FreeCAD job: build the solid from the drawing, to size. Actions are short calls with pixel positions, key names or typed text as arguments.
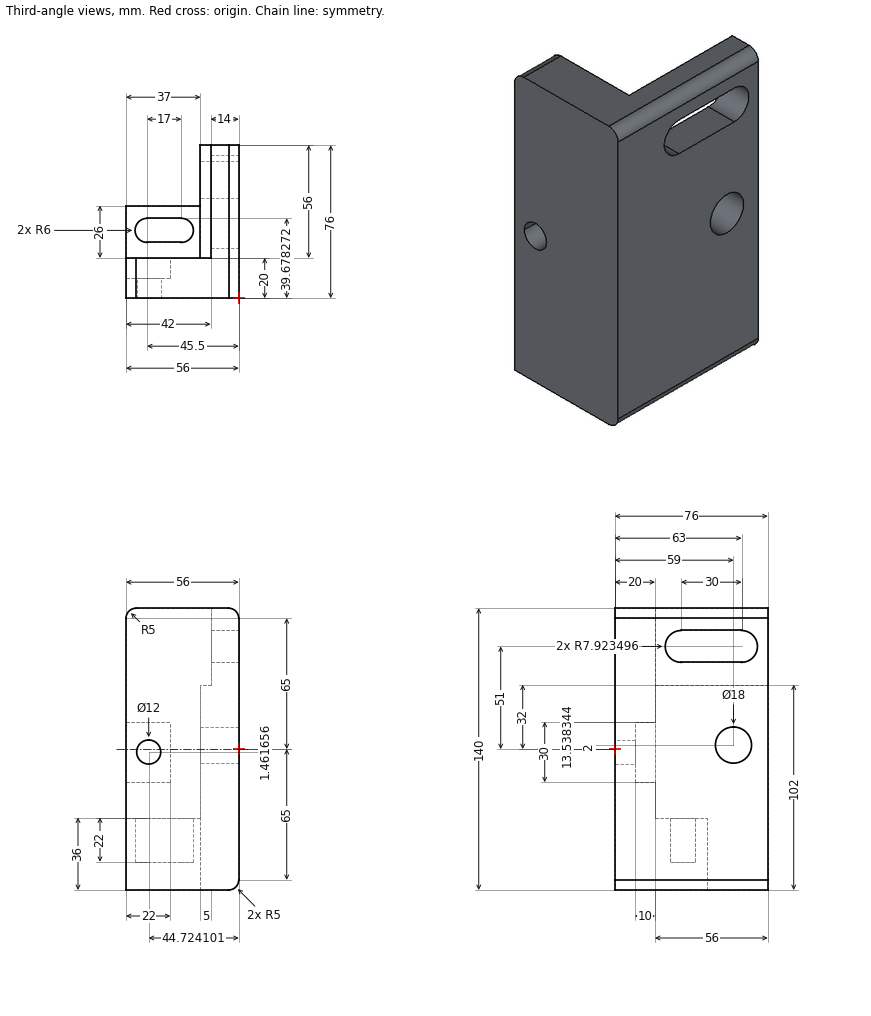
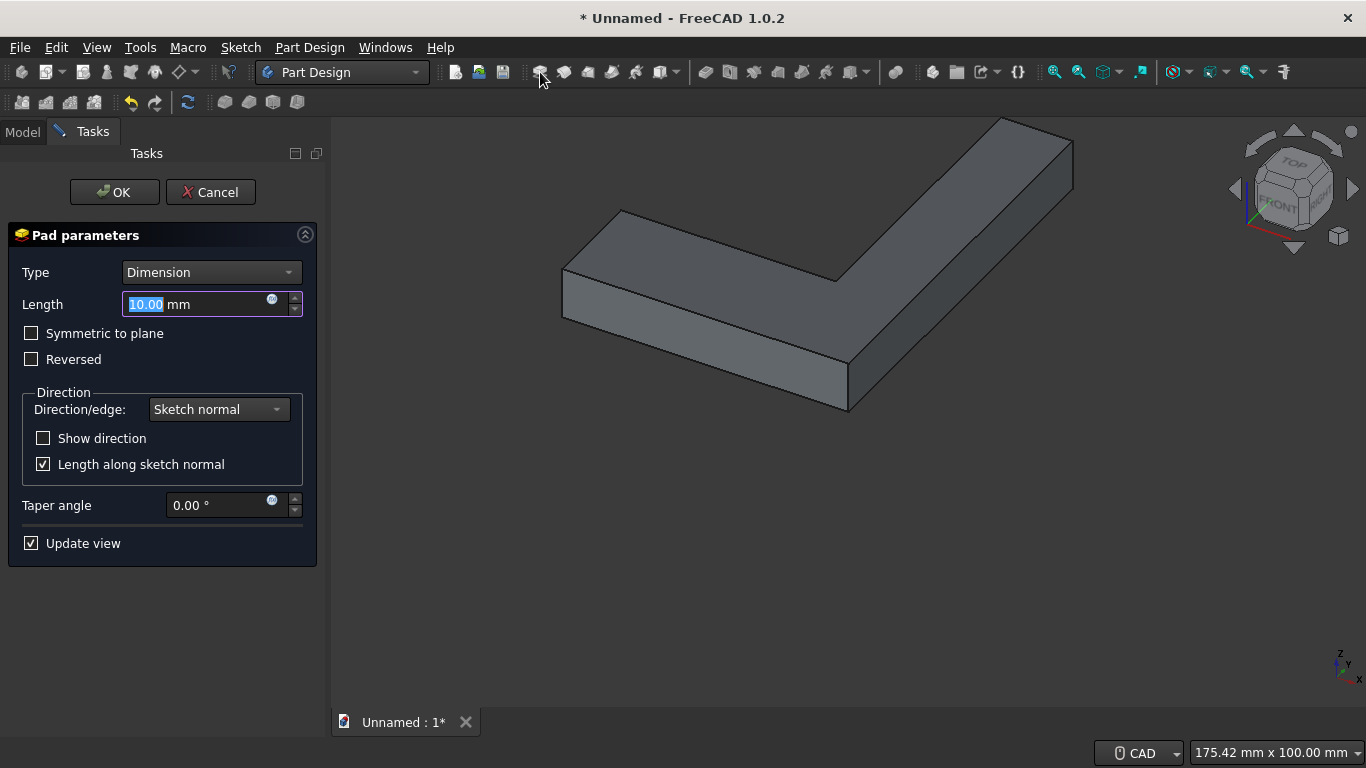
text(140)
key(Tab)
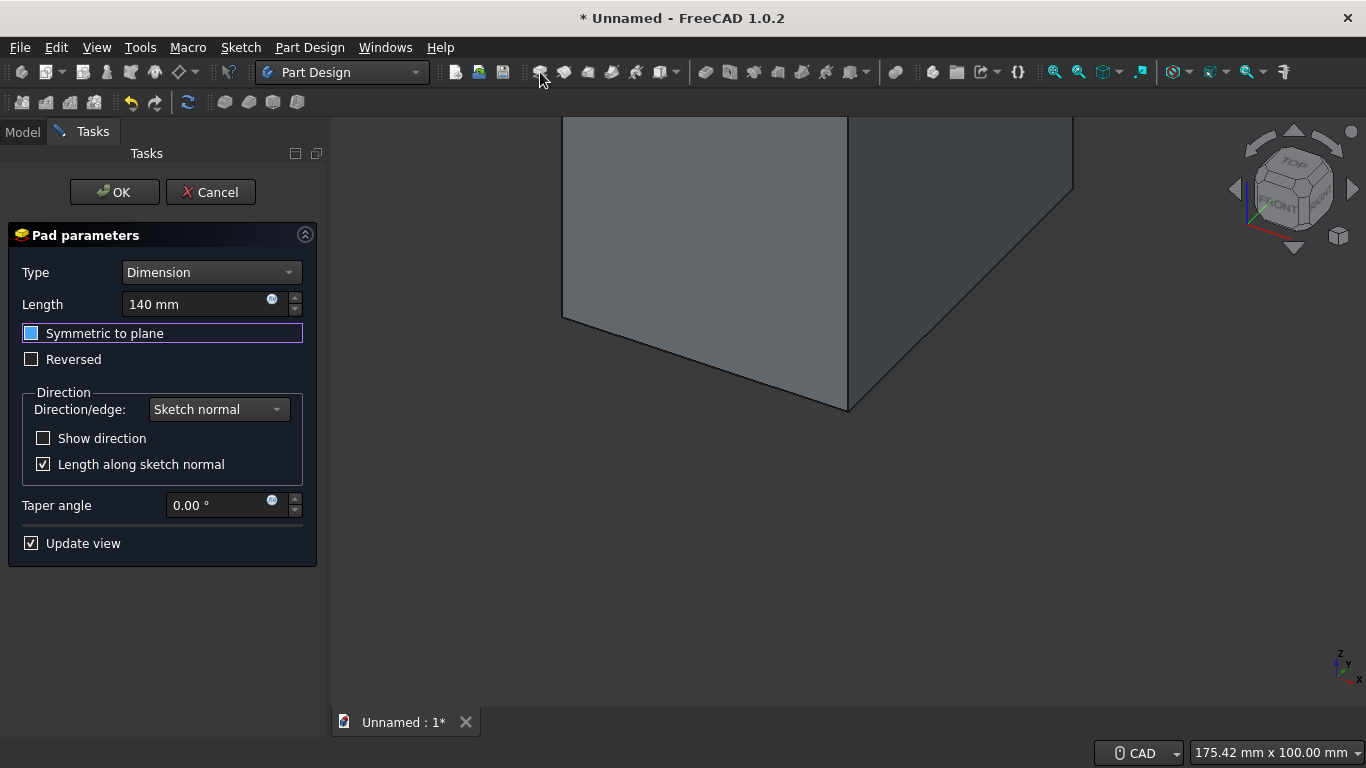
click(30, 333)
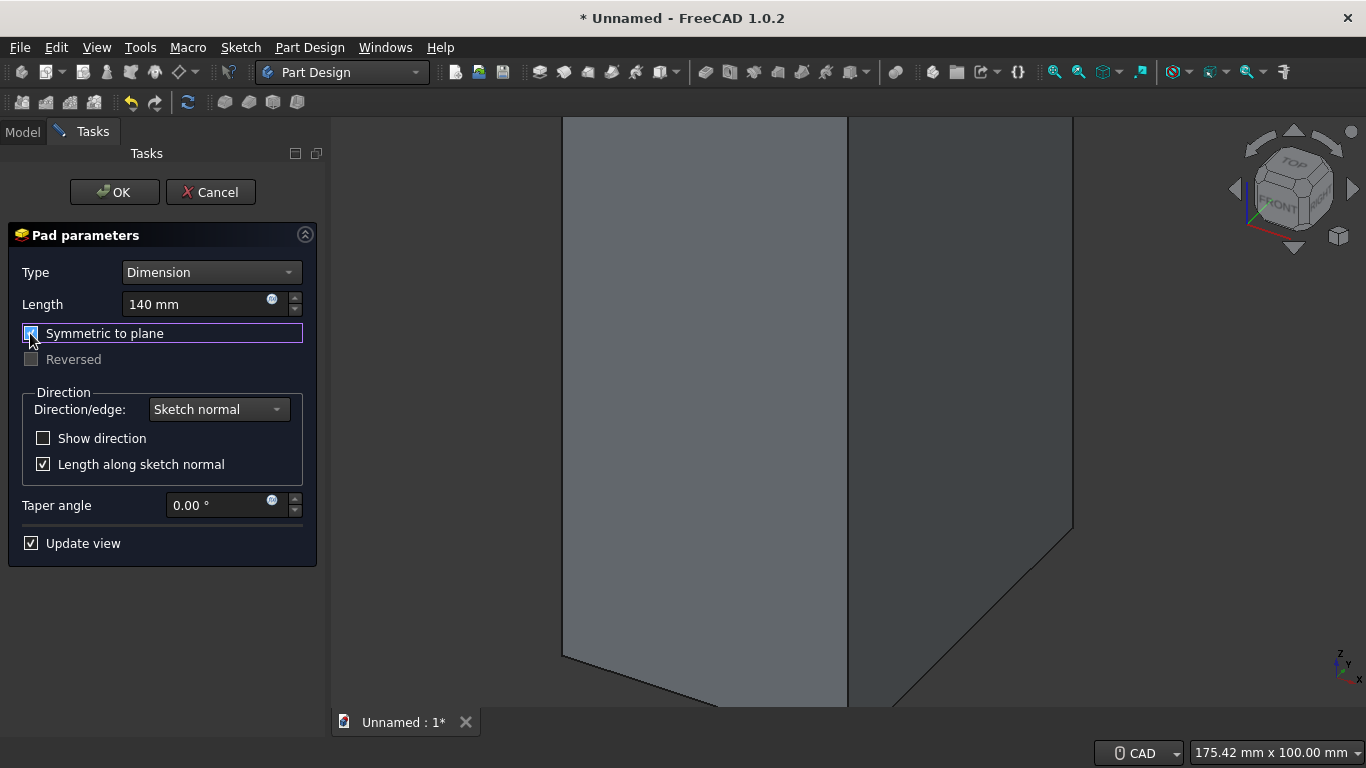
click(115, 192)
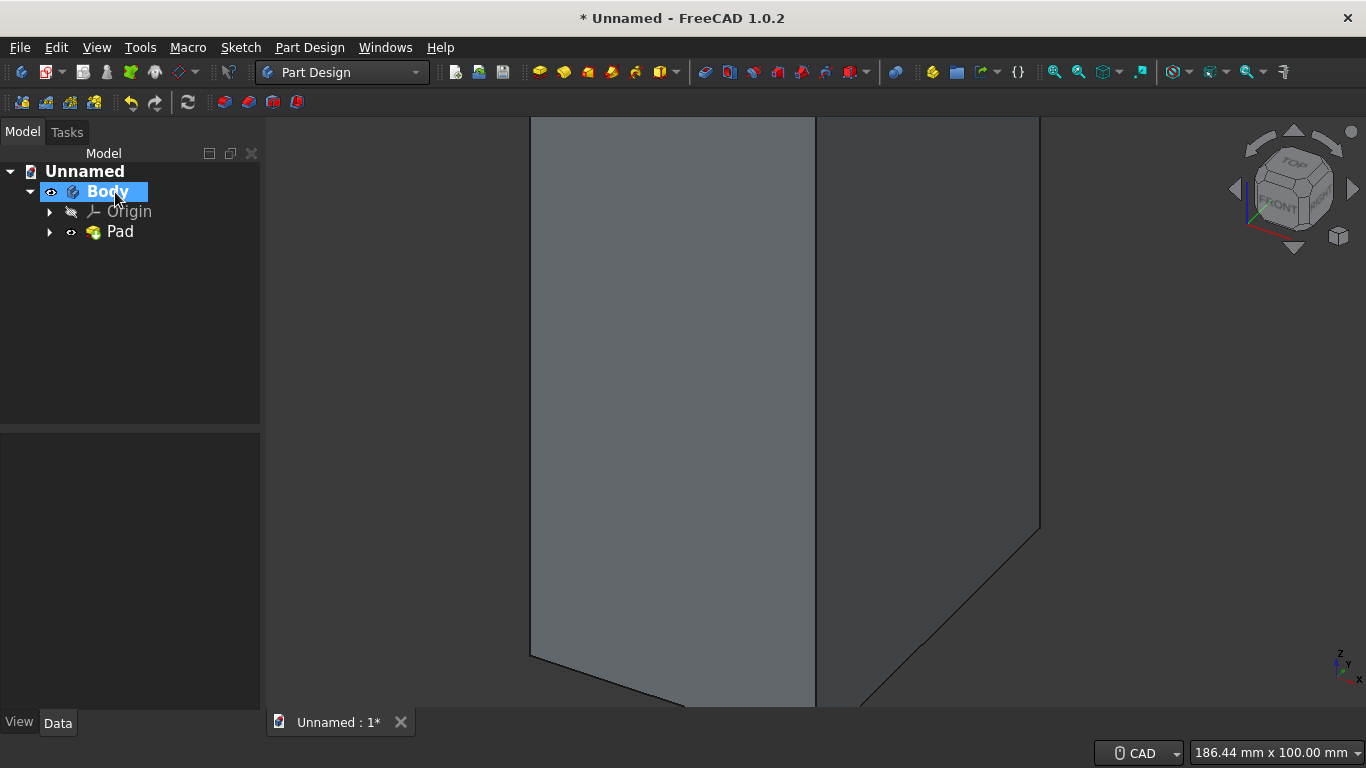
key(v)
key(f)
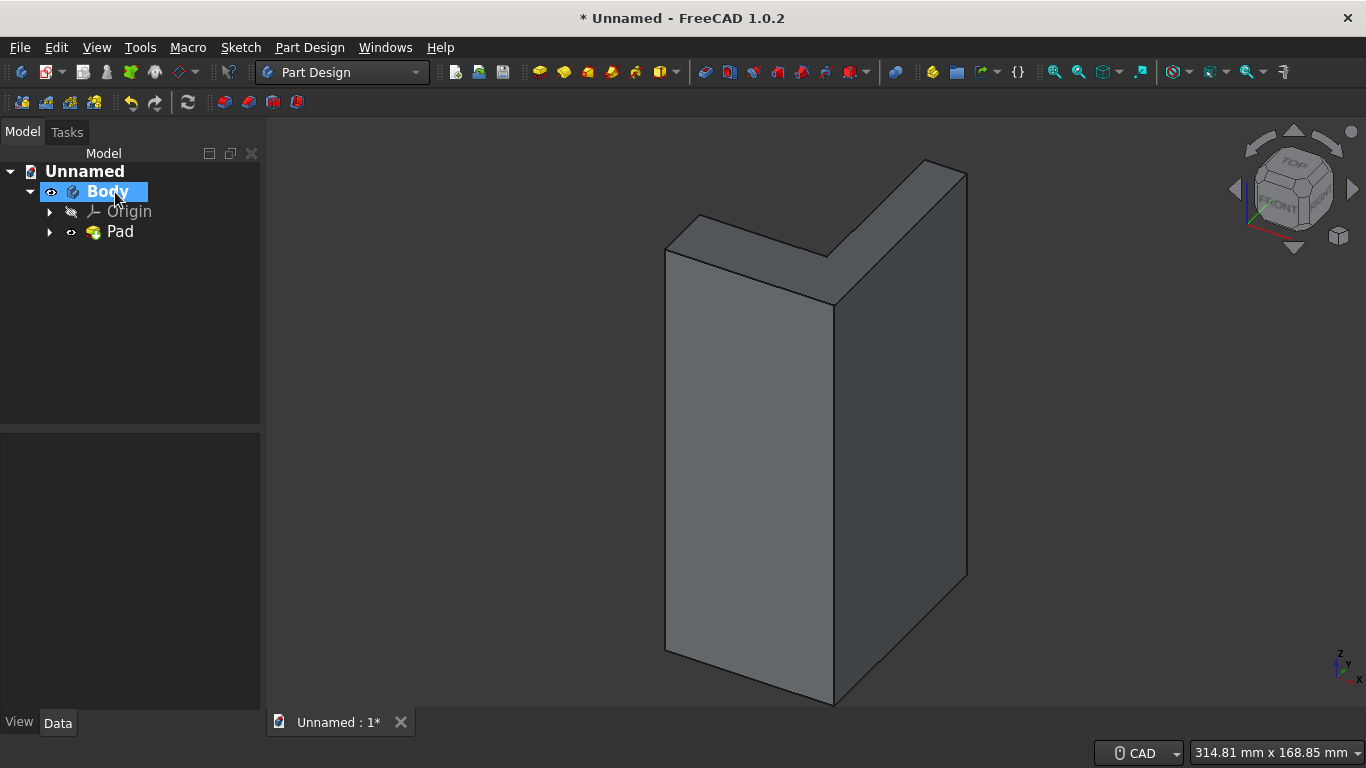
key(4)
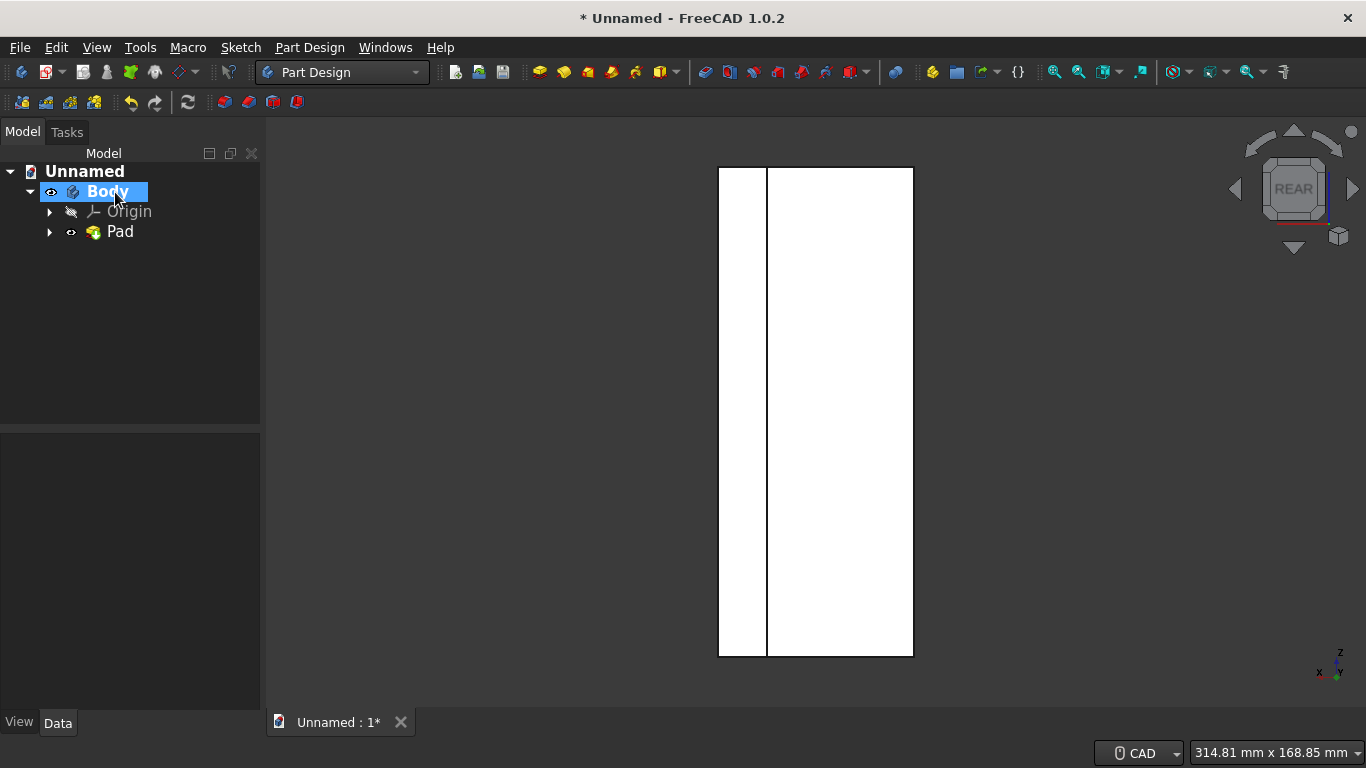
click(743, 201)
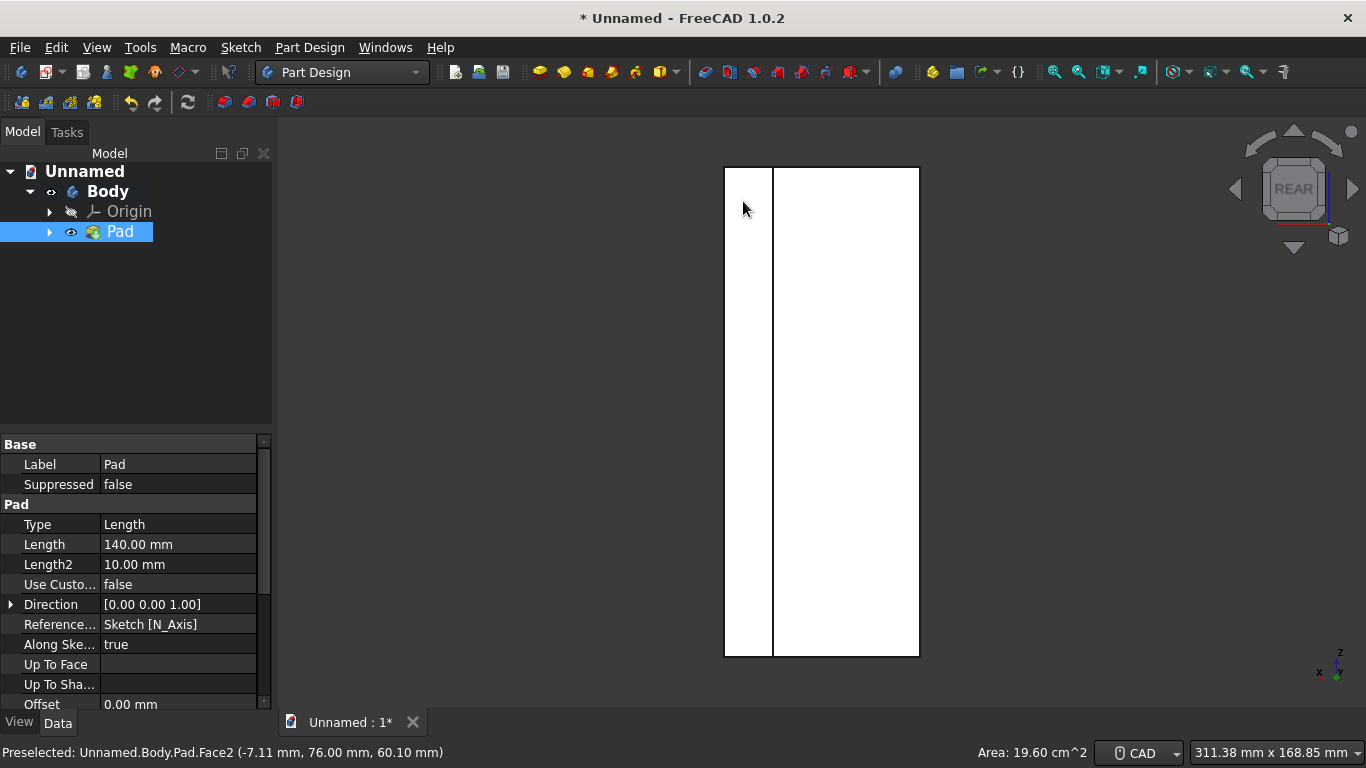
click(46, 72)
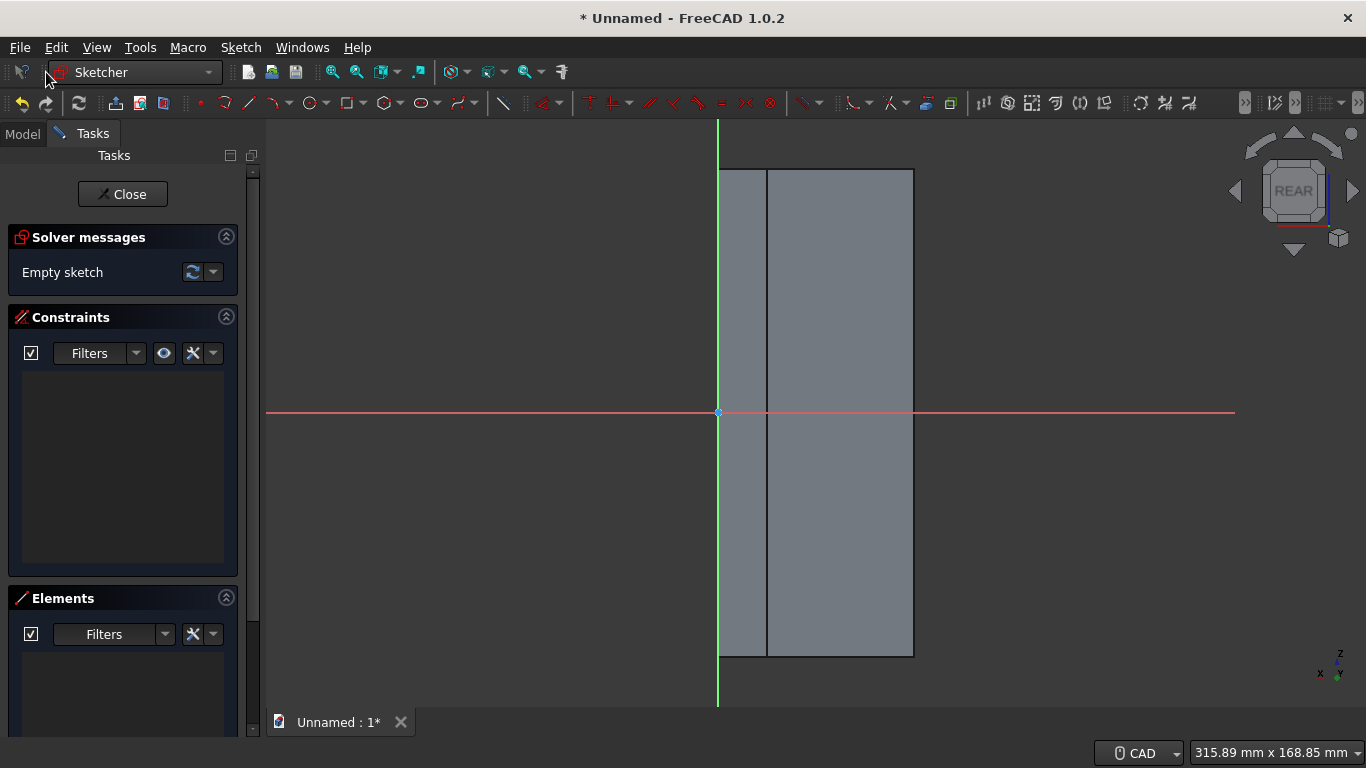
scroll(839, 413, down, 1)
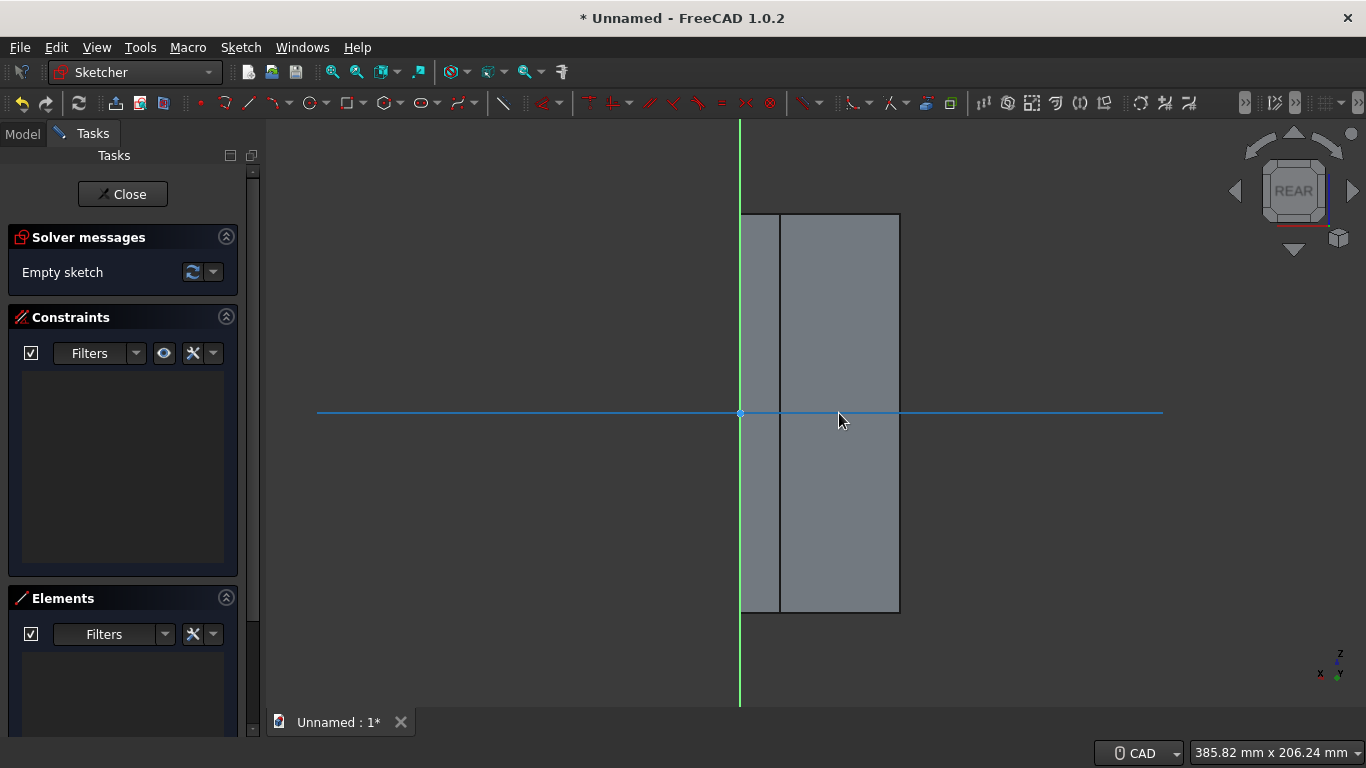
key(g)
key(m)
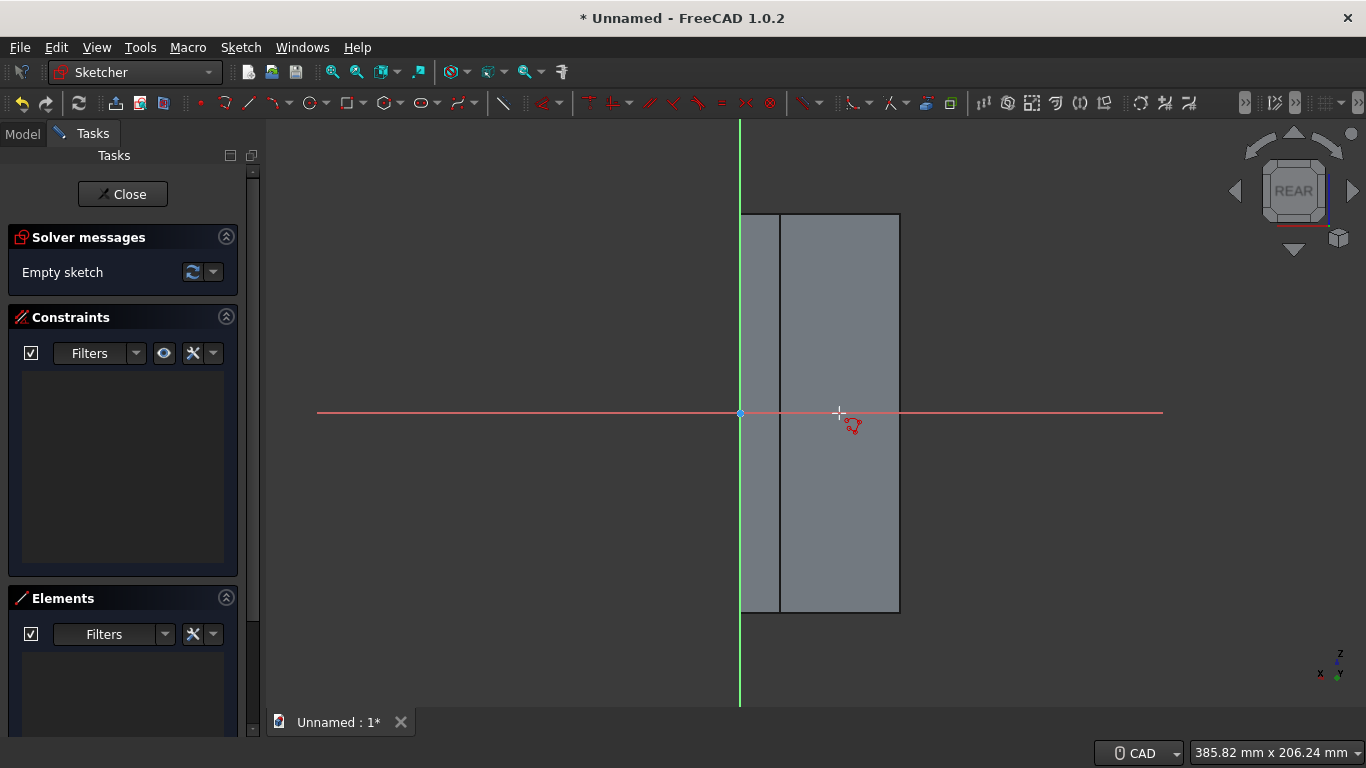
click(740, 598)
click(749, 613)
click(755, 613)
right_click(755, 613)